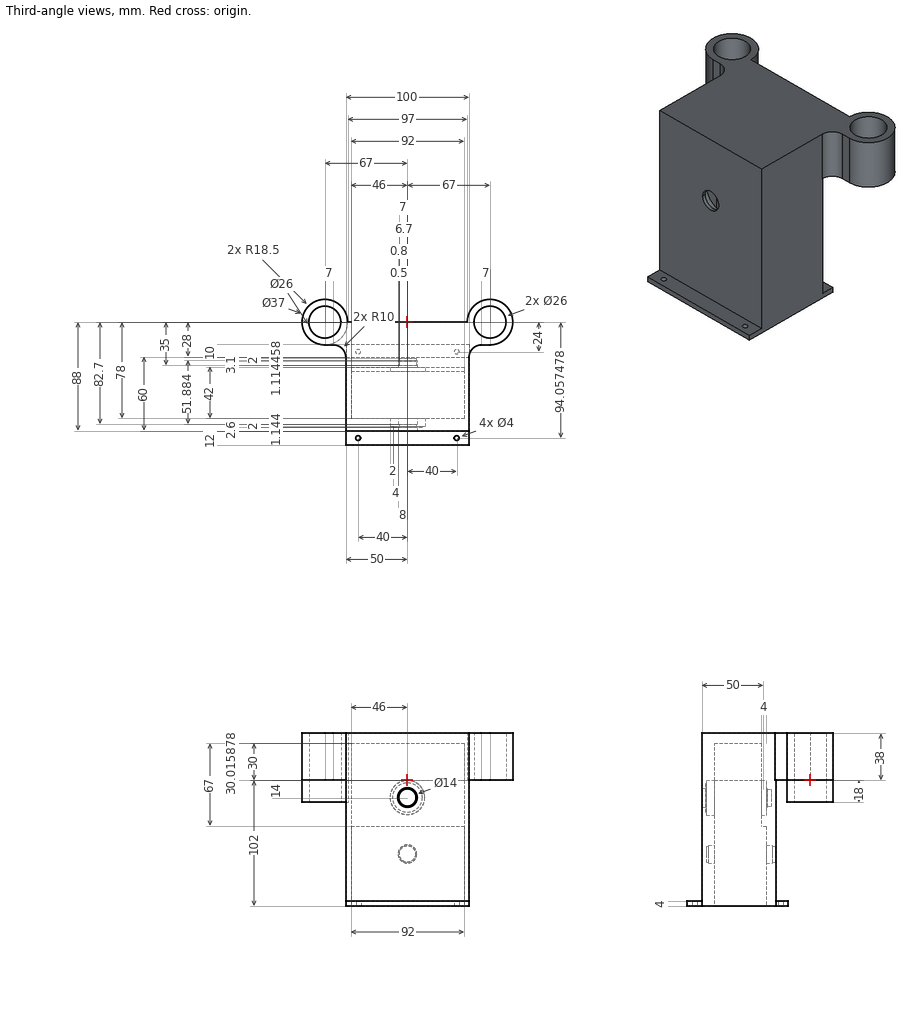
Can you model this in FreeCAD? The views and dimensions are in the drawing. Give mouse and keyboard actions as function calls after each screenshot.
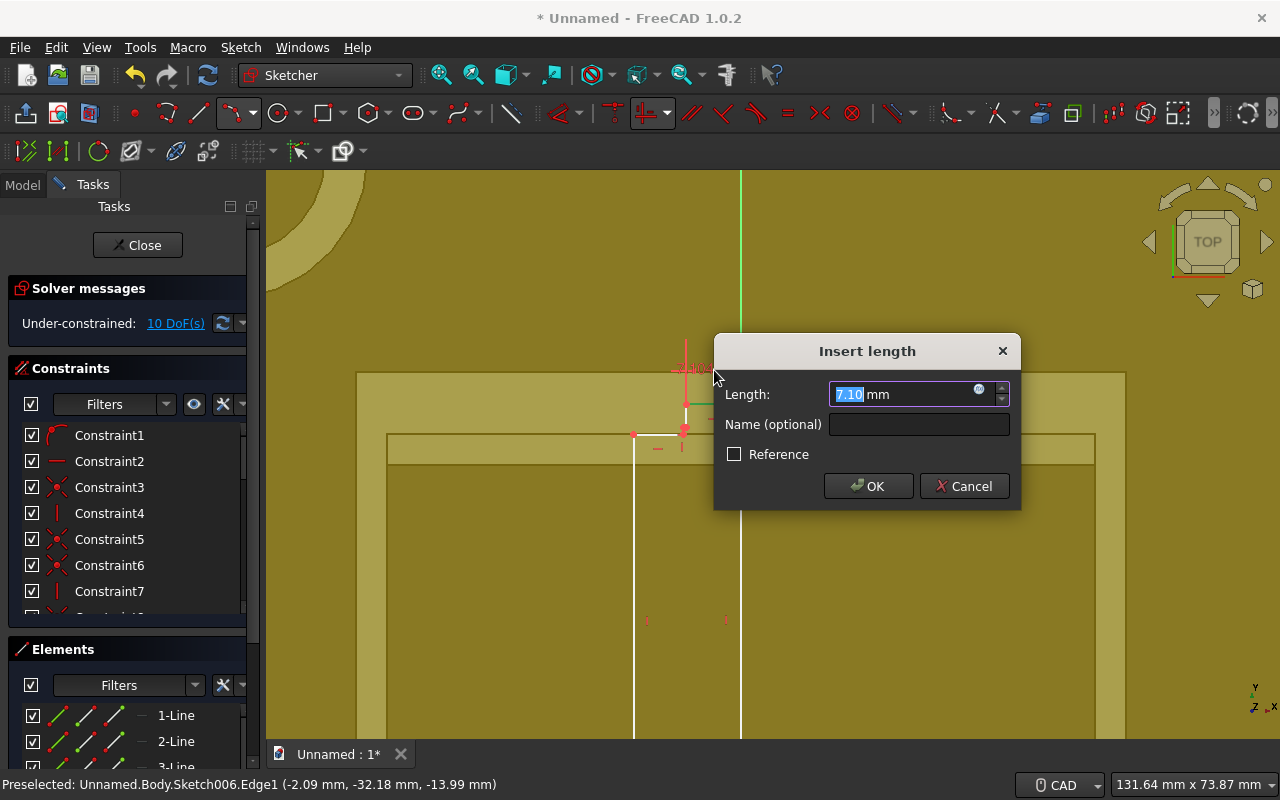
text(7)
key(Return)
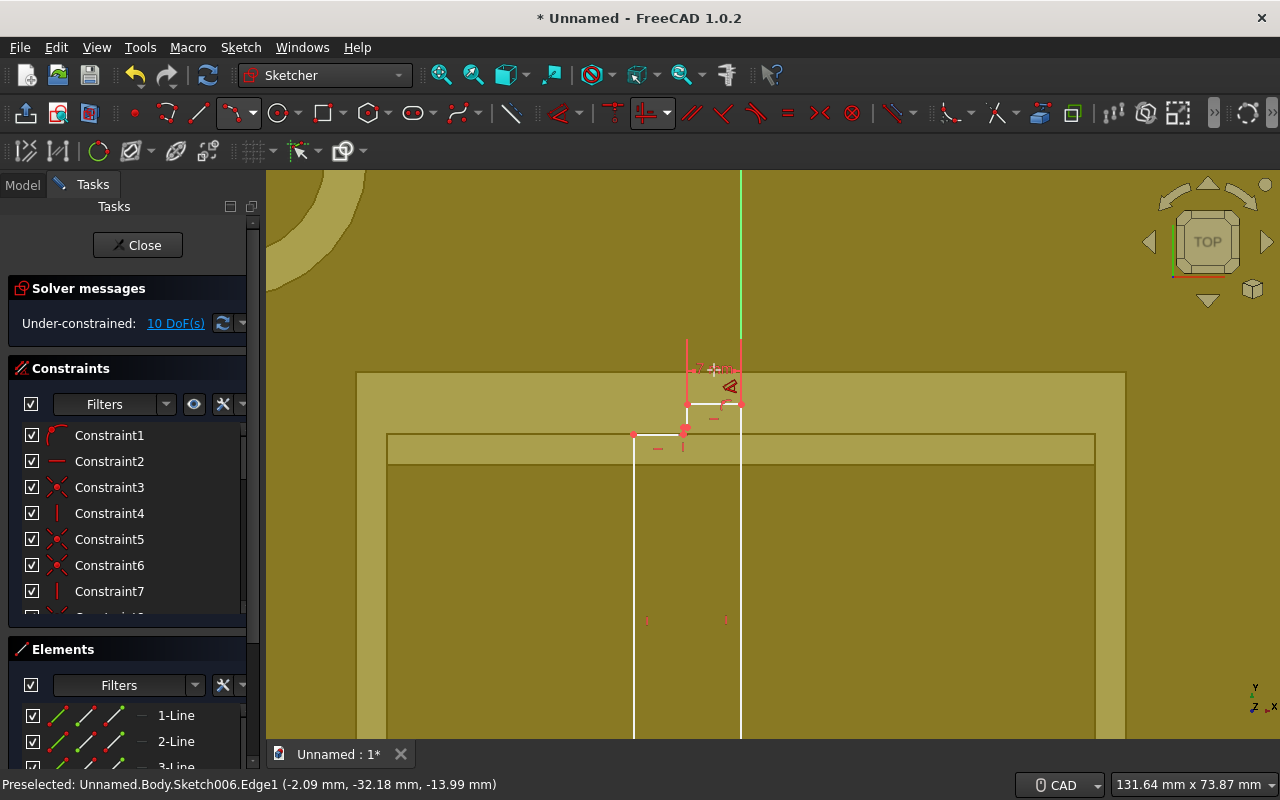
scroll(726, 405, down, 3)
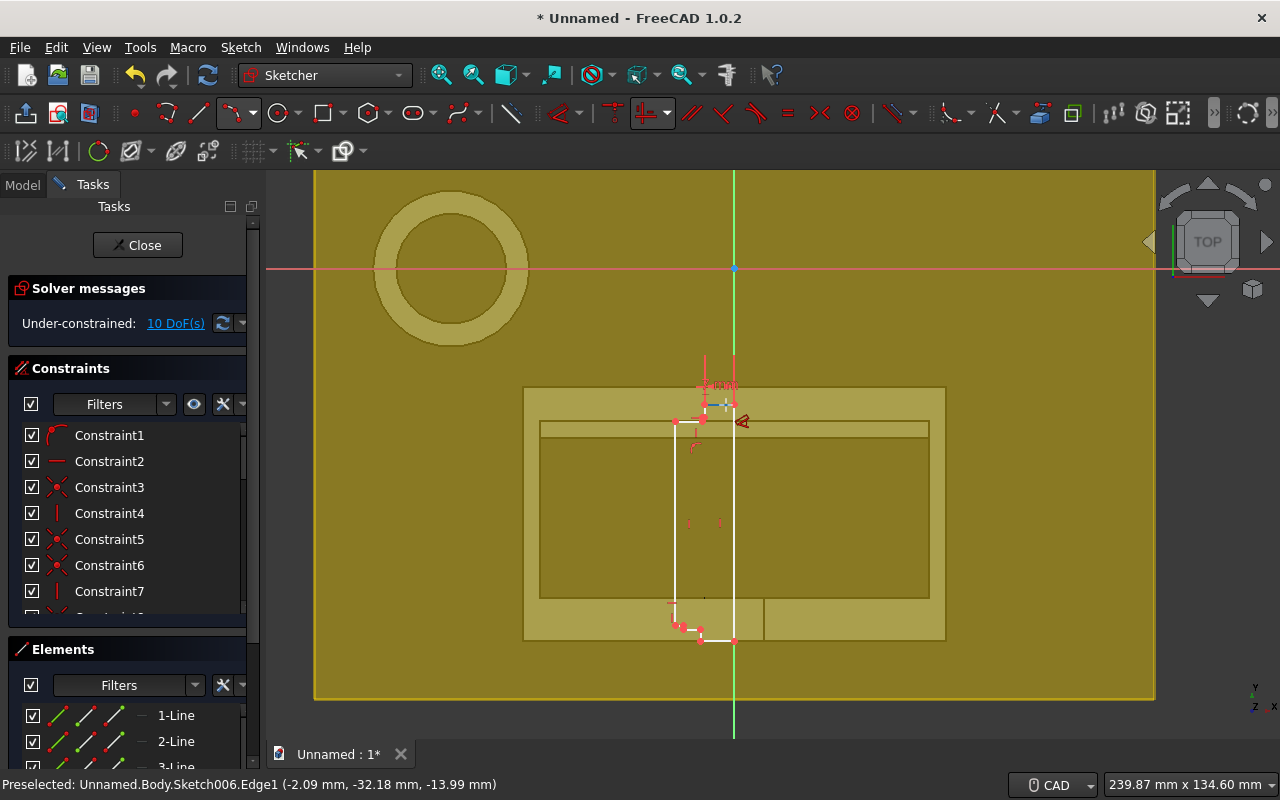
scroll(680, 626, up, 8)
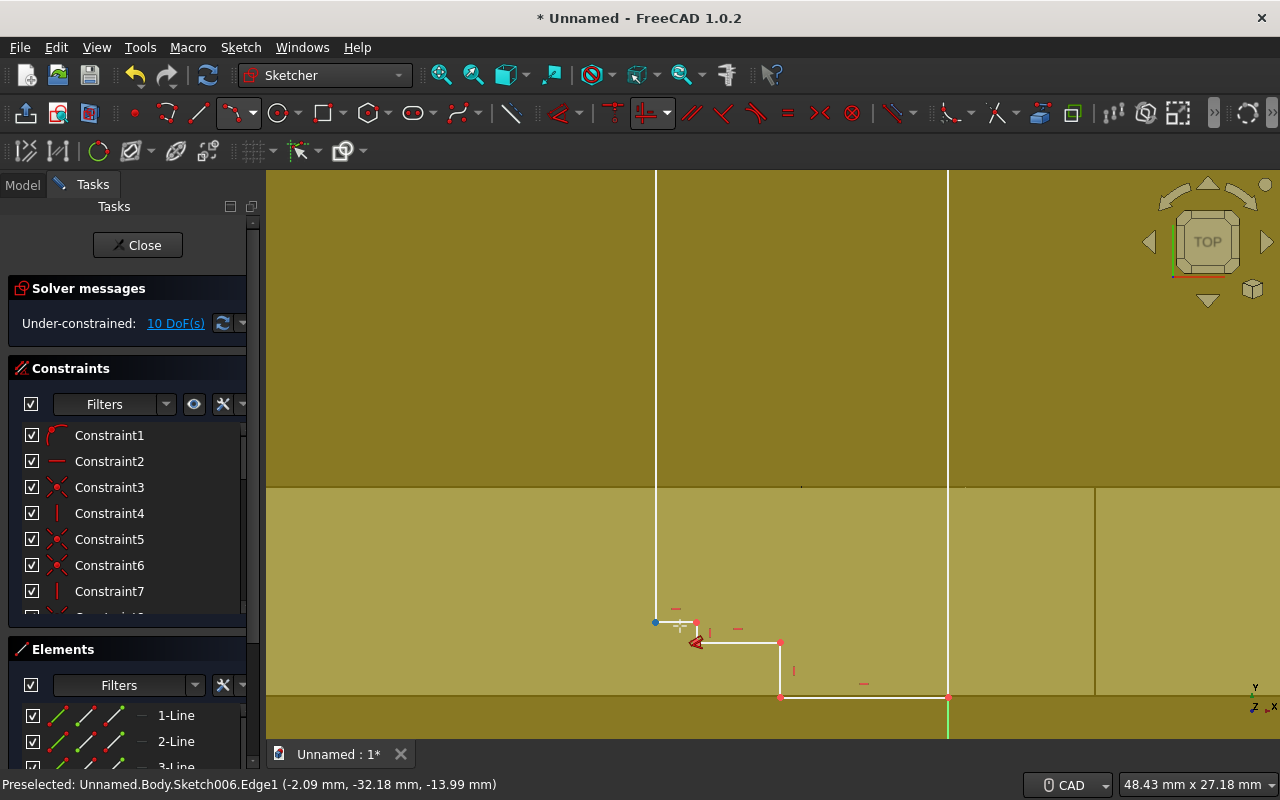
click(676, 622)
click(676, 656)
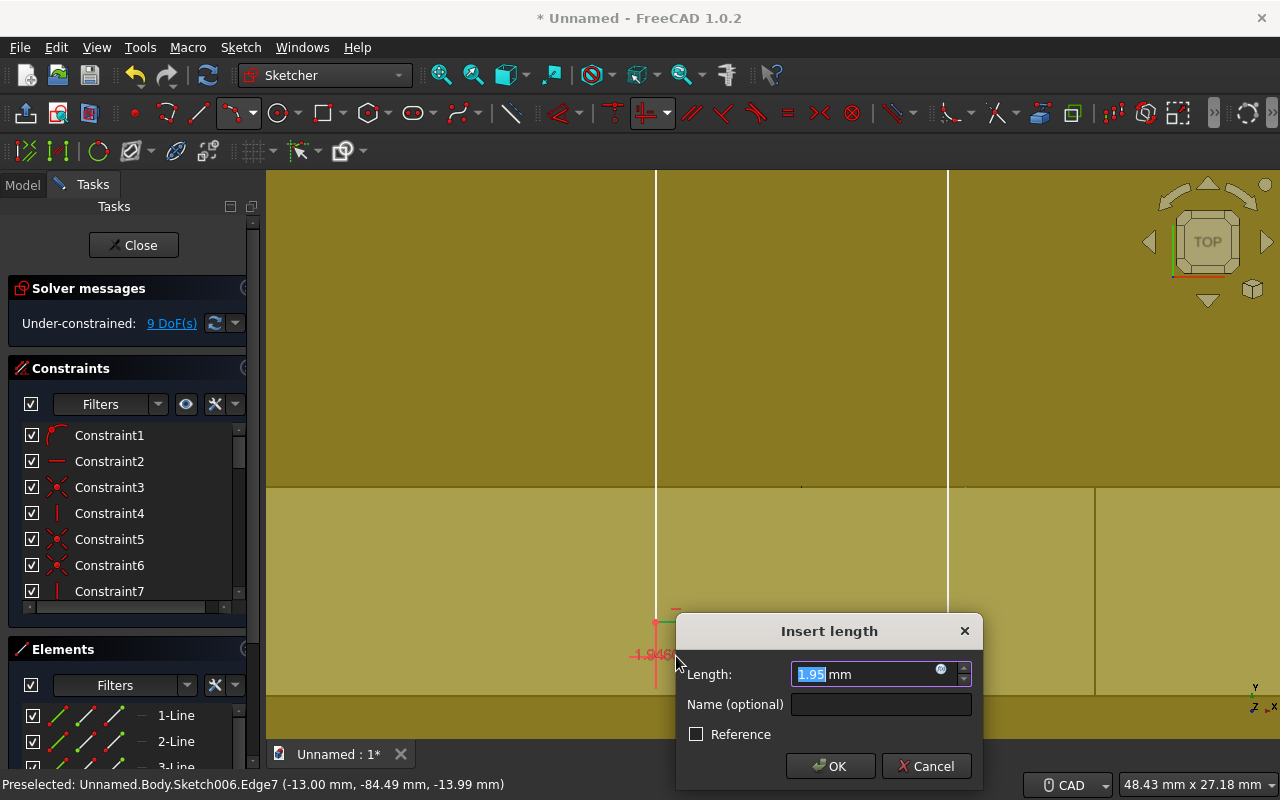
text(2)
key(Return)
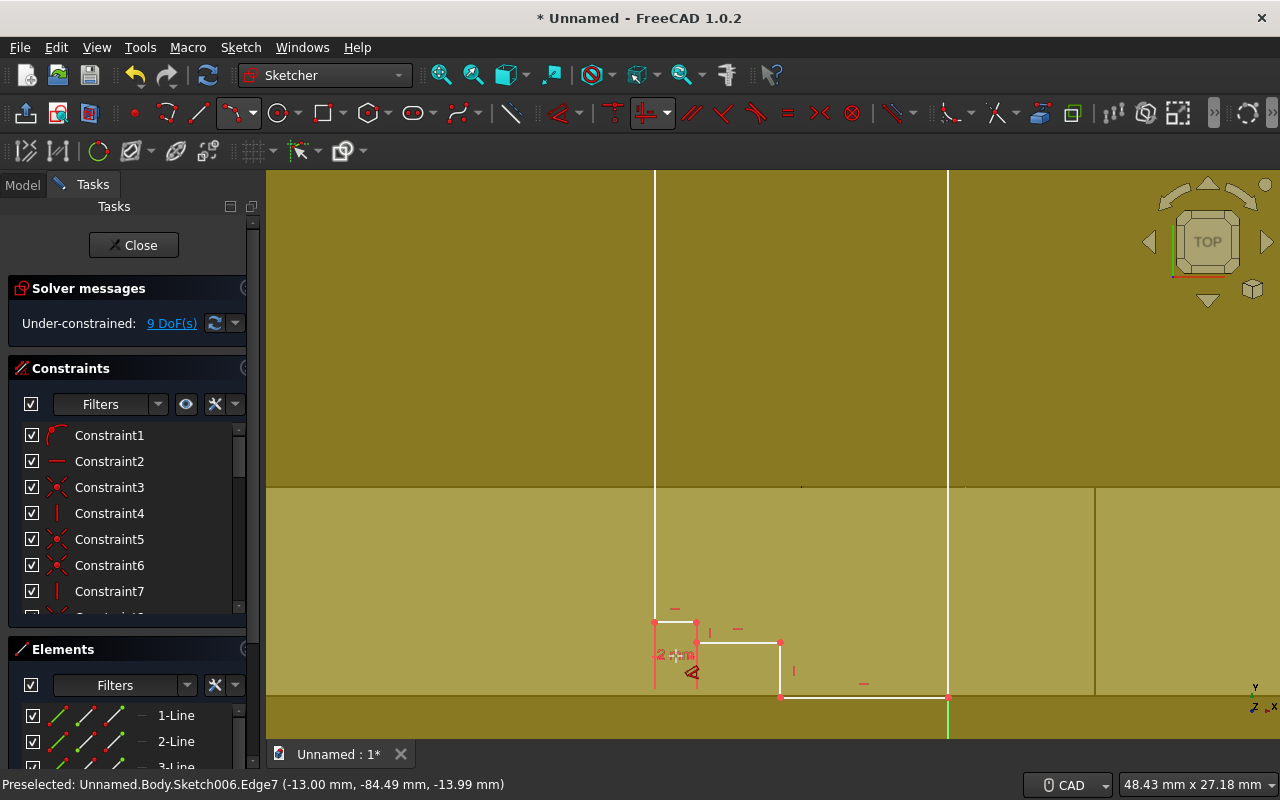
click(722, 642)
click(739, 676)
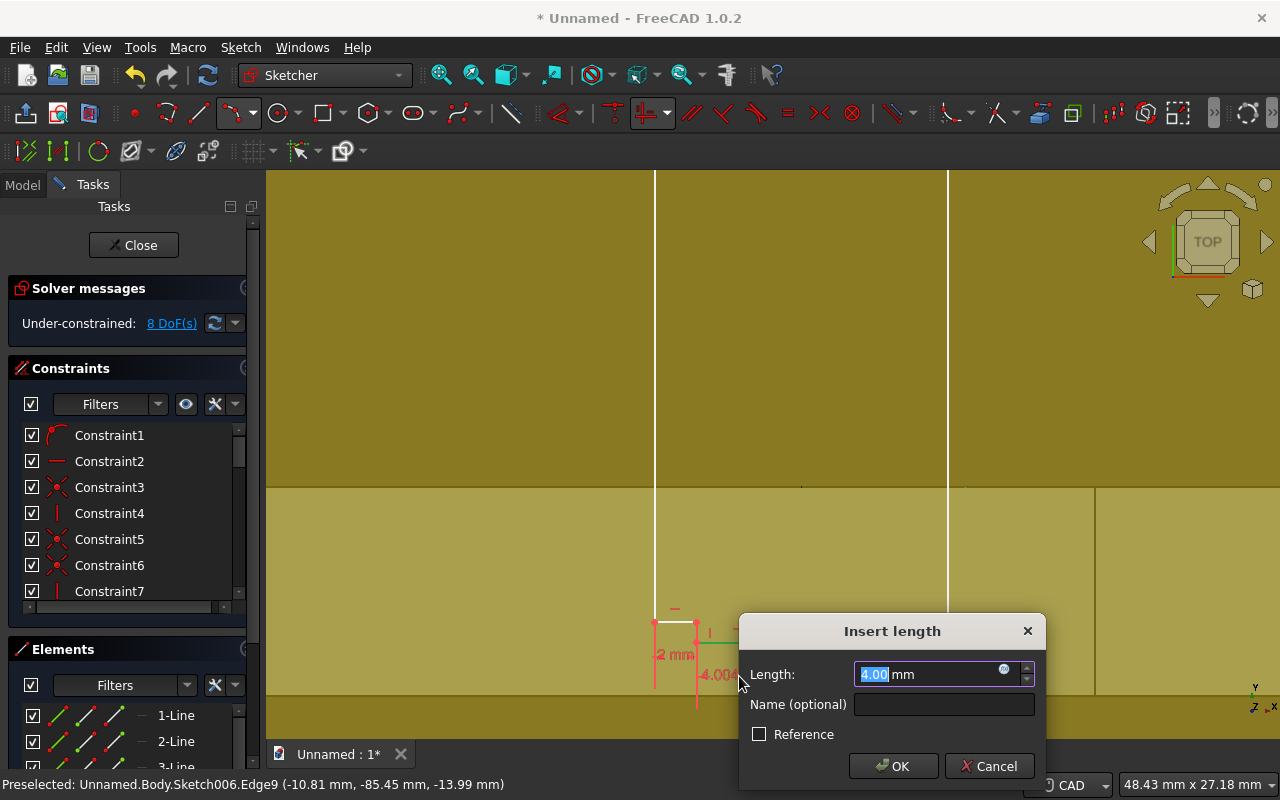
text(4)
key(Return)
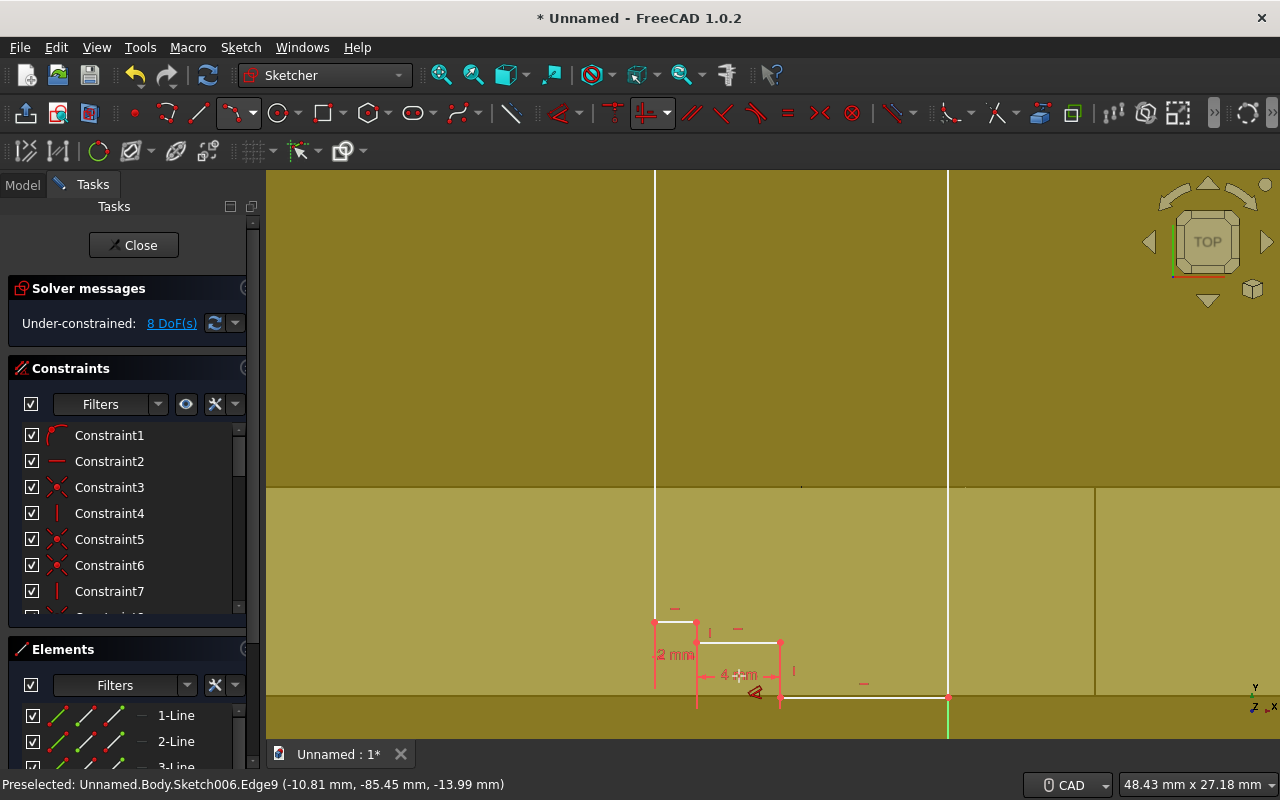
scroll(680, 626, down, 8)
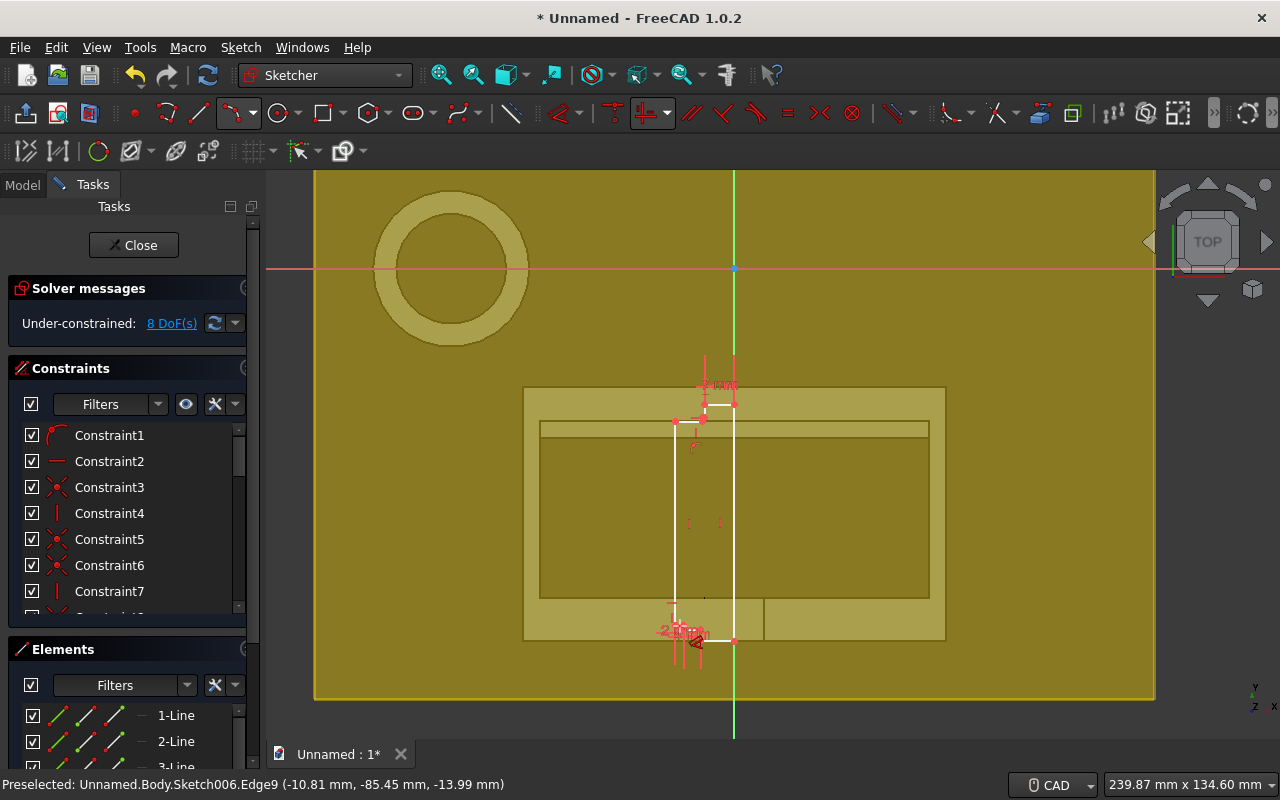
scroll(711, 641, up, 2)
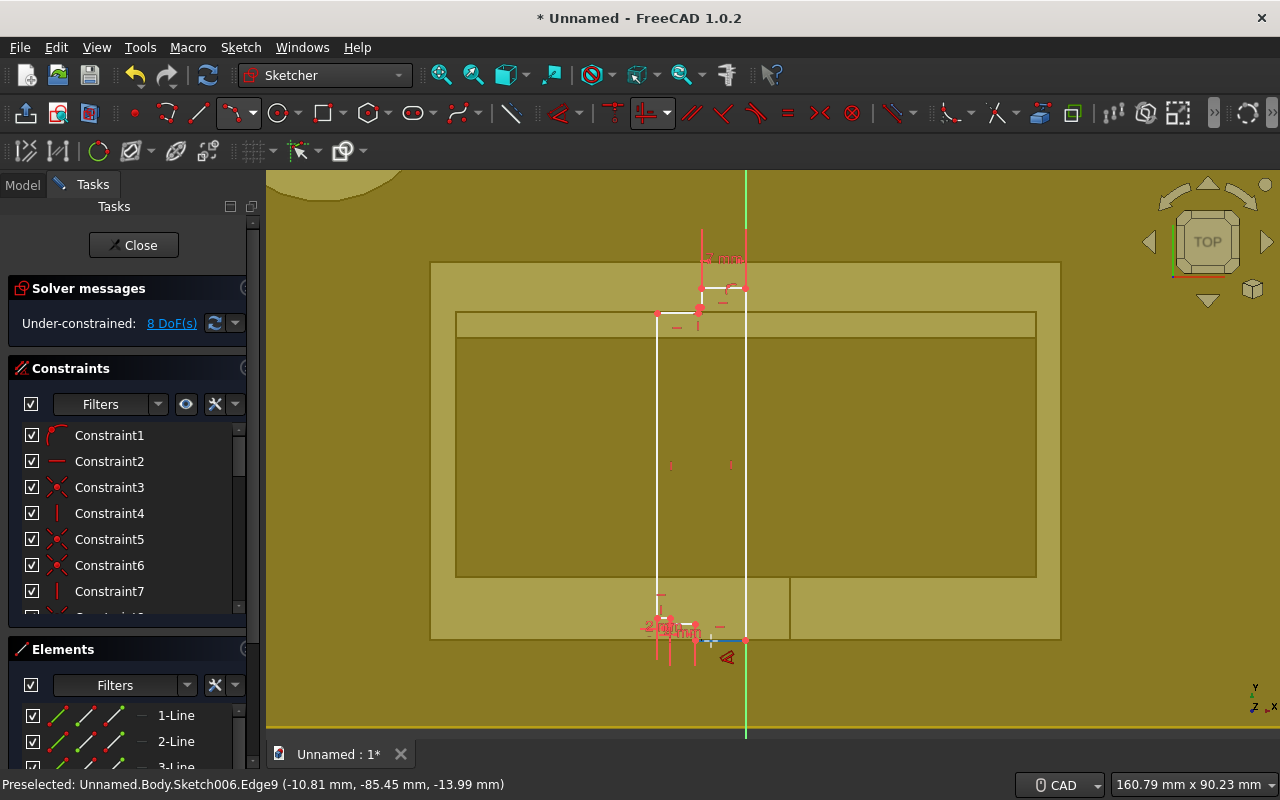
click(710, 641)
click(721, 675)